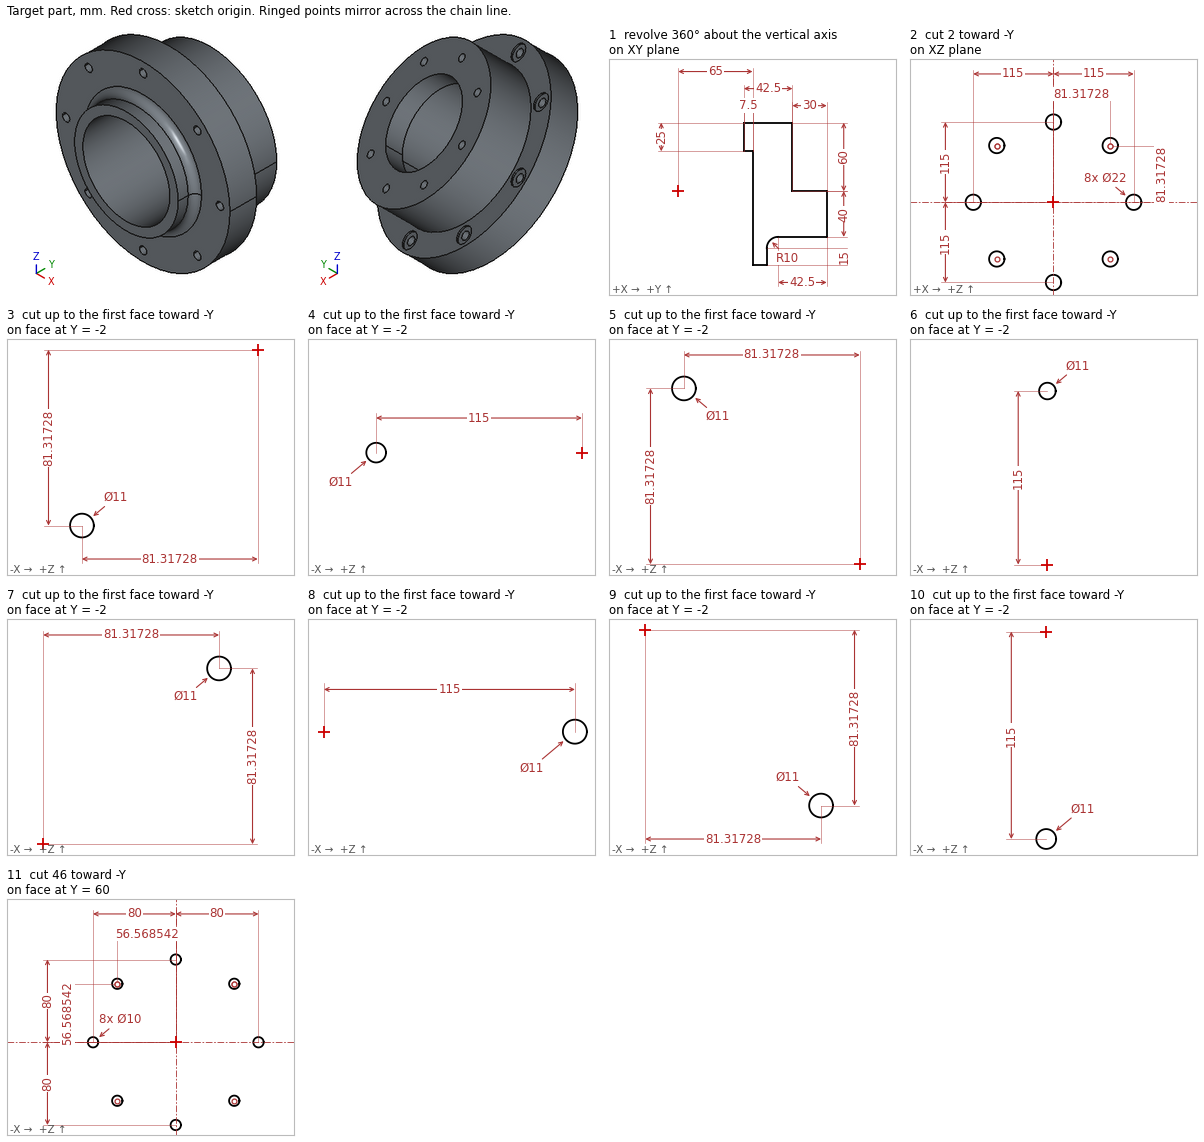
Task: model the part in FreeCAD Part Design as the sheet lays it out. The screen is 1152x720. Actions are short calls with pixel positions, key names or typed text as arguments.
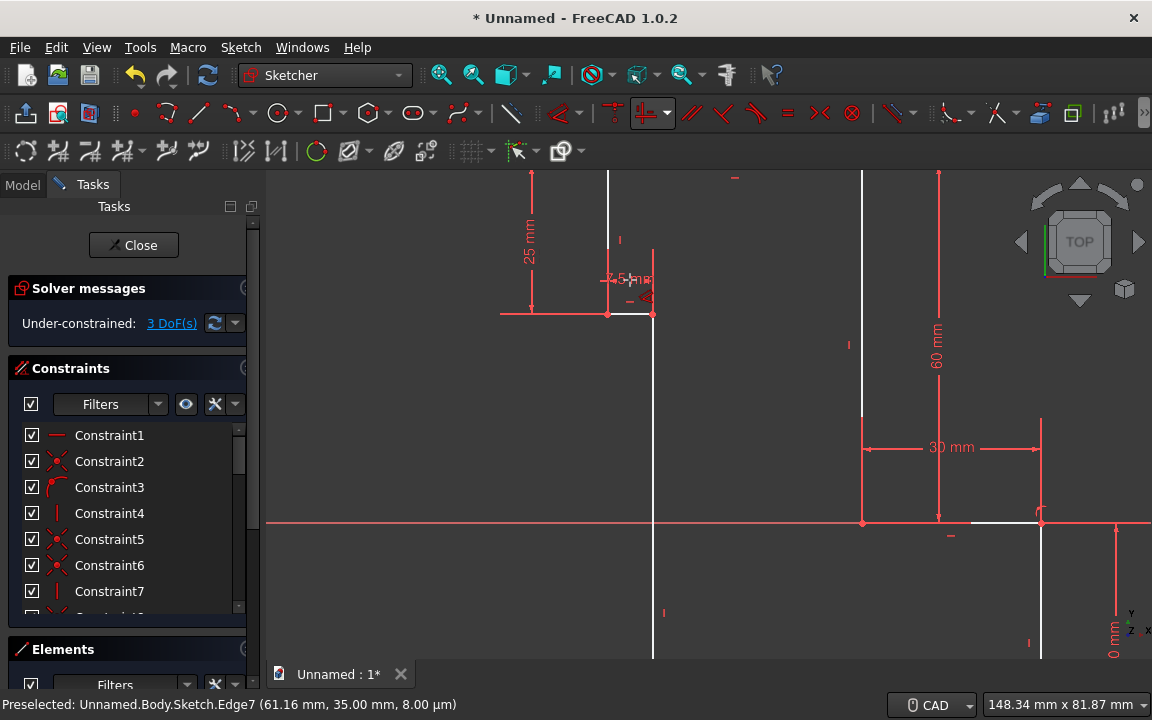
click(653, 314)
click(473, 280)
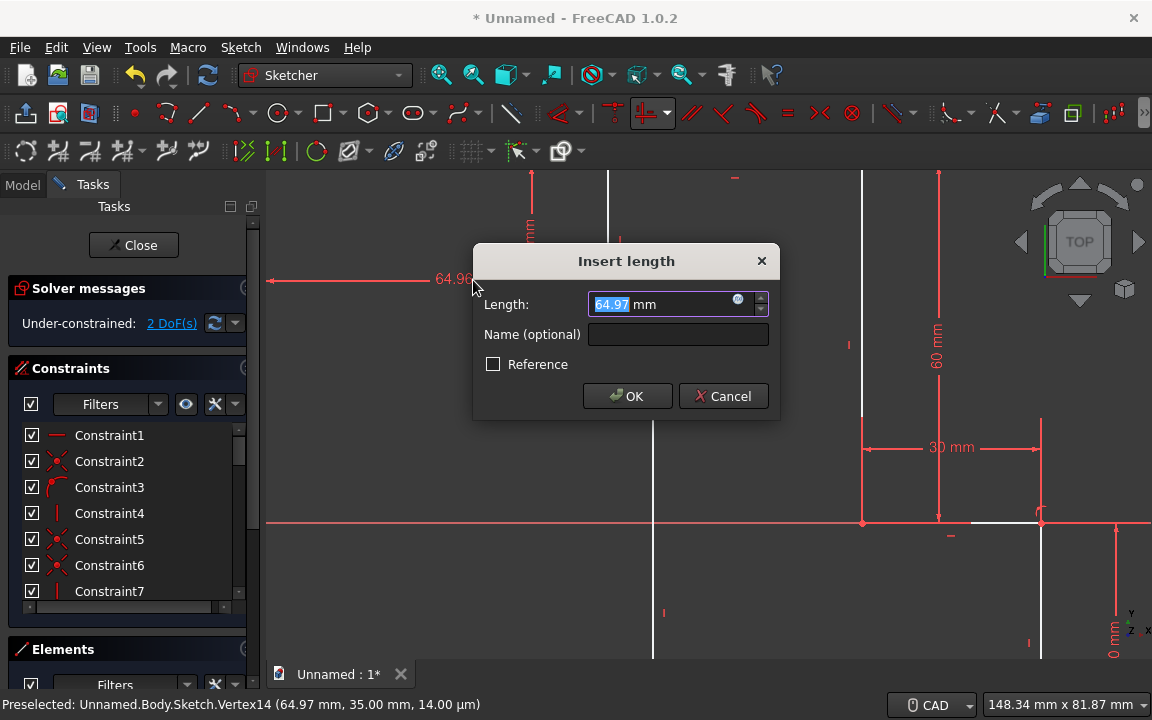
text(65)
key(Return)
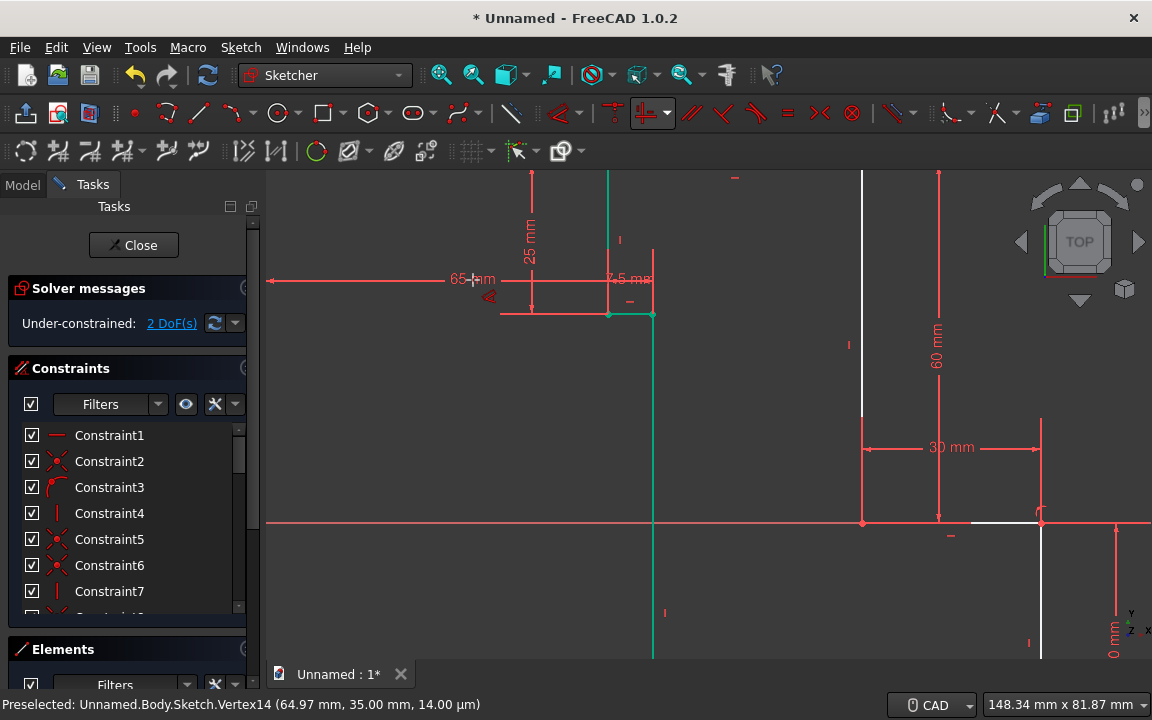
scroll(630, 314, down, 4)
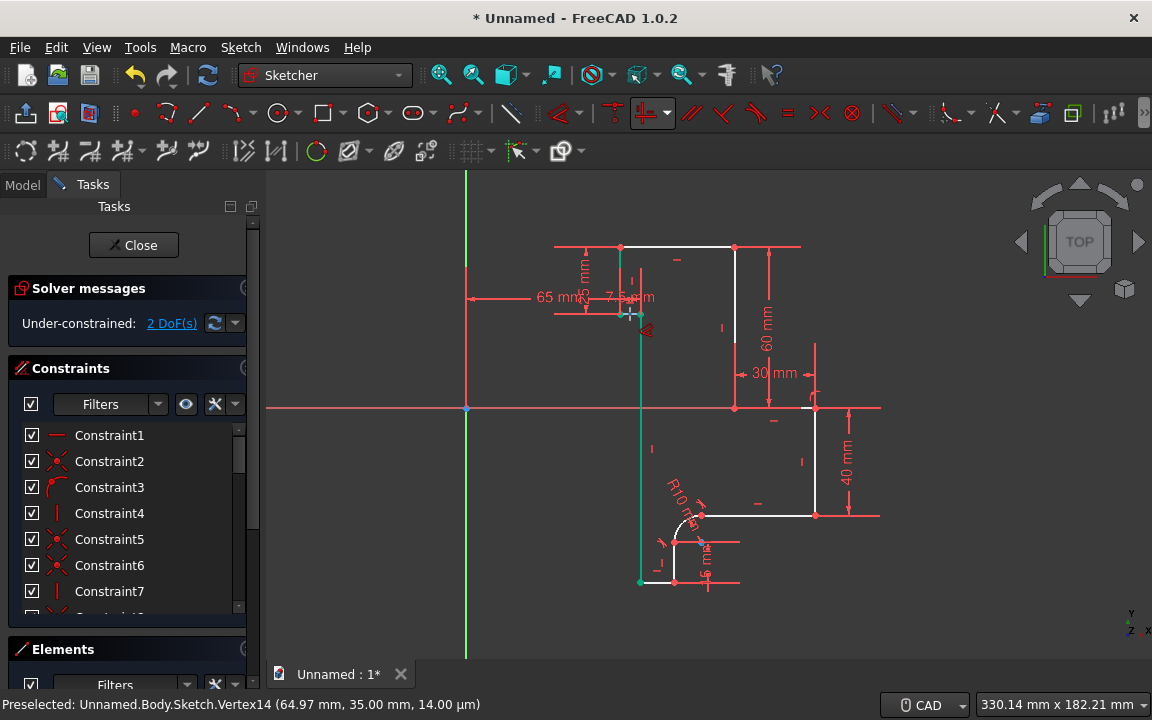
click(735, 516)
click(784, 550)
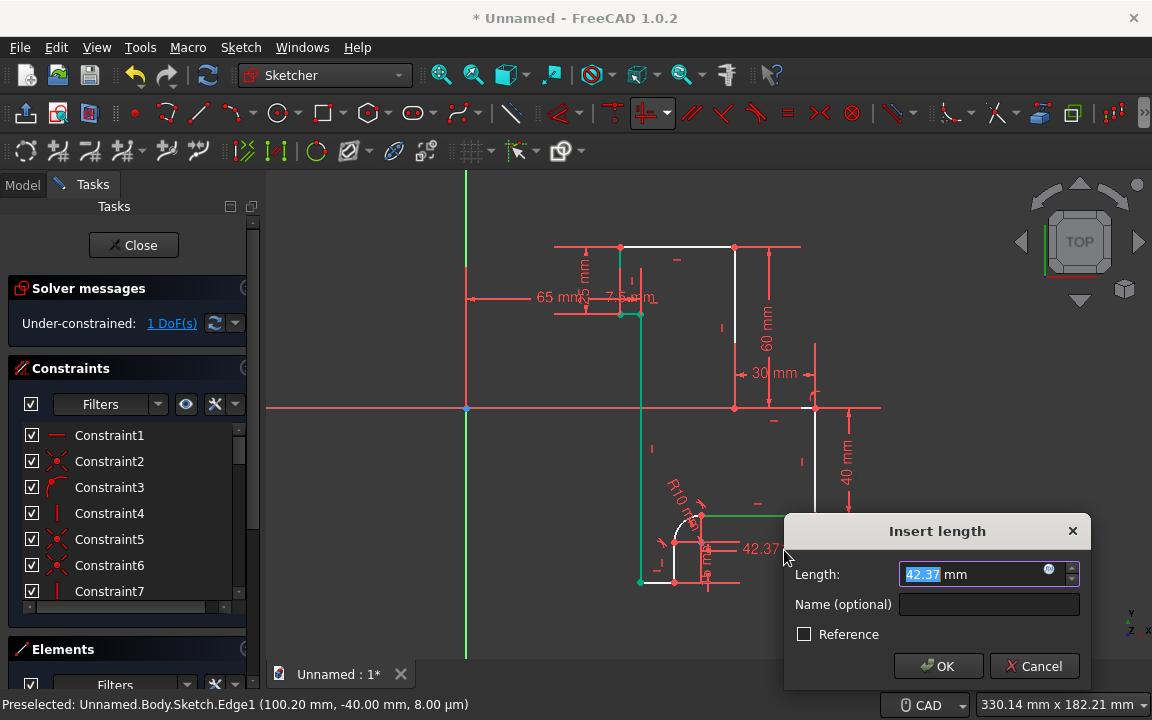
text(42.5)
key(Return)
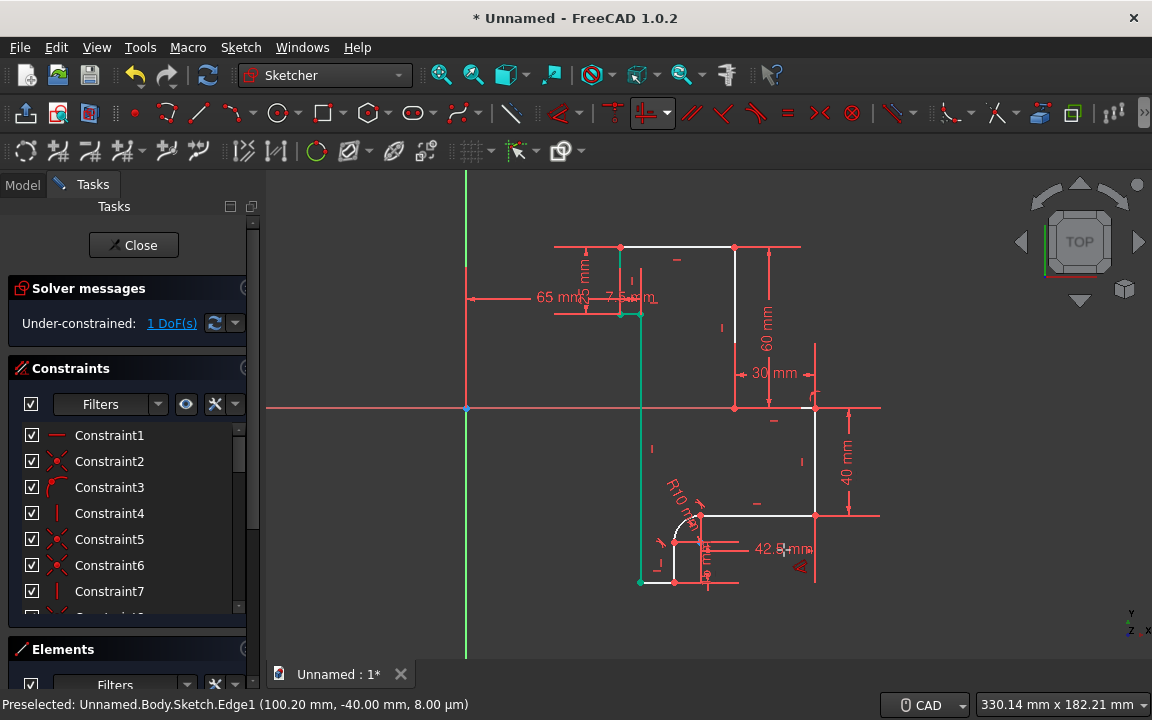
click(700, 247)
click(677, 213)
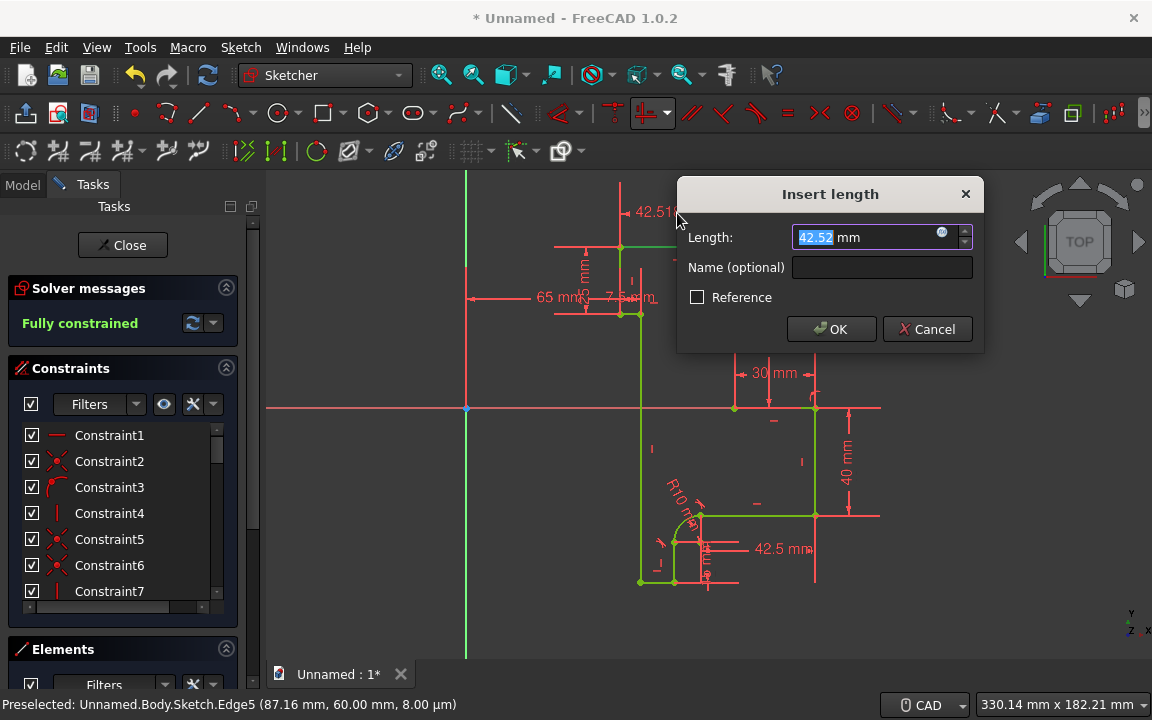
text(42.5)
key(Return)
key(Escape)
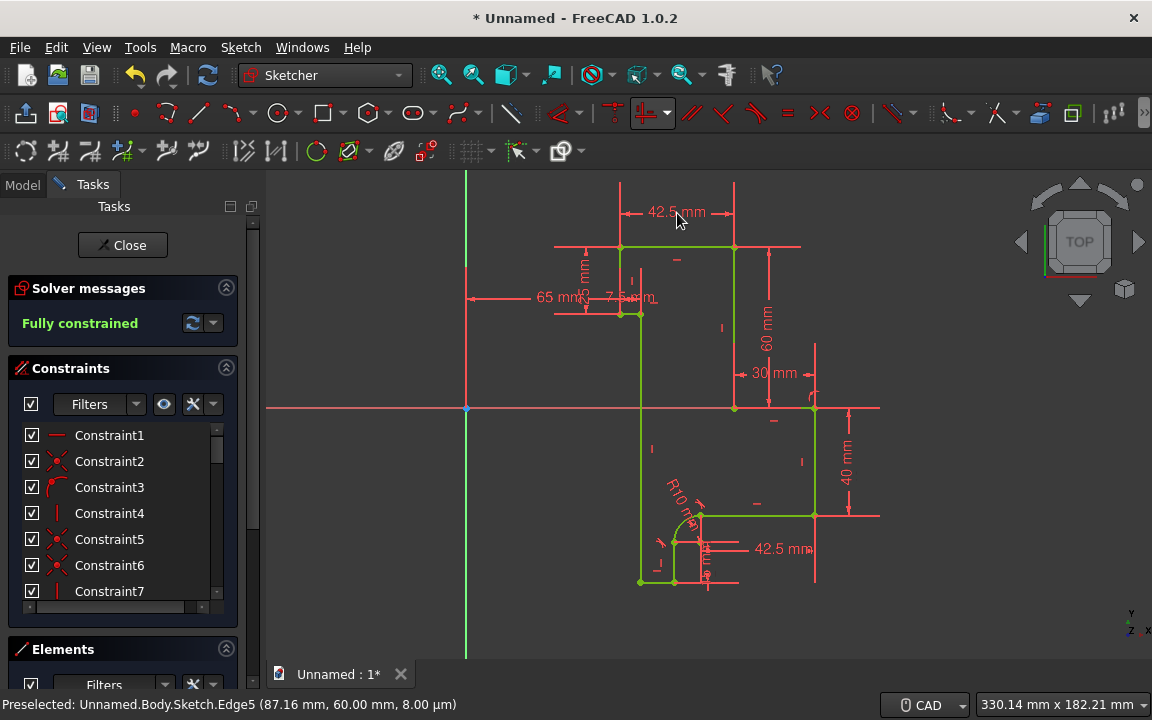
click(123, 245)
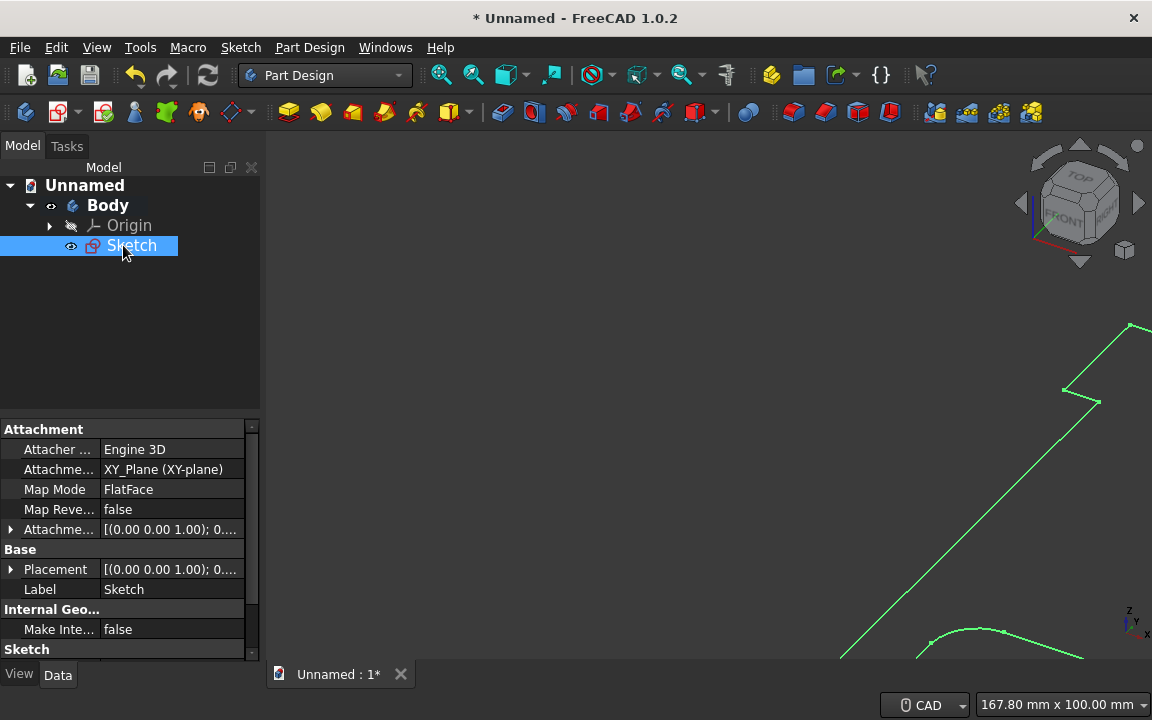
click(322, 112)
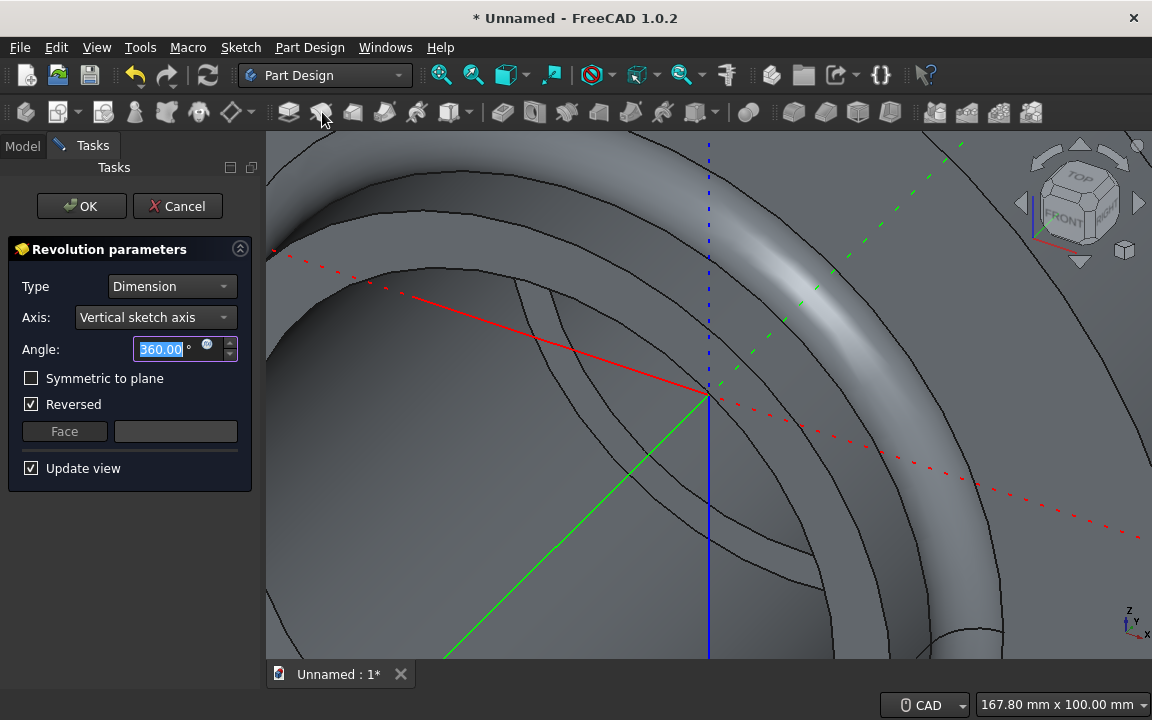
click(82, 206)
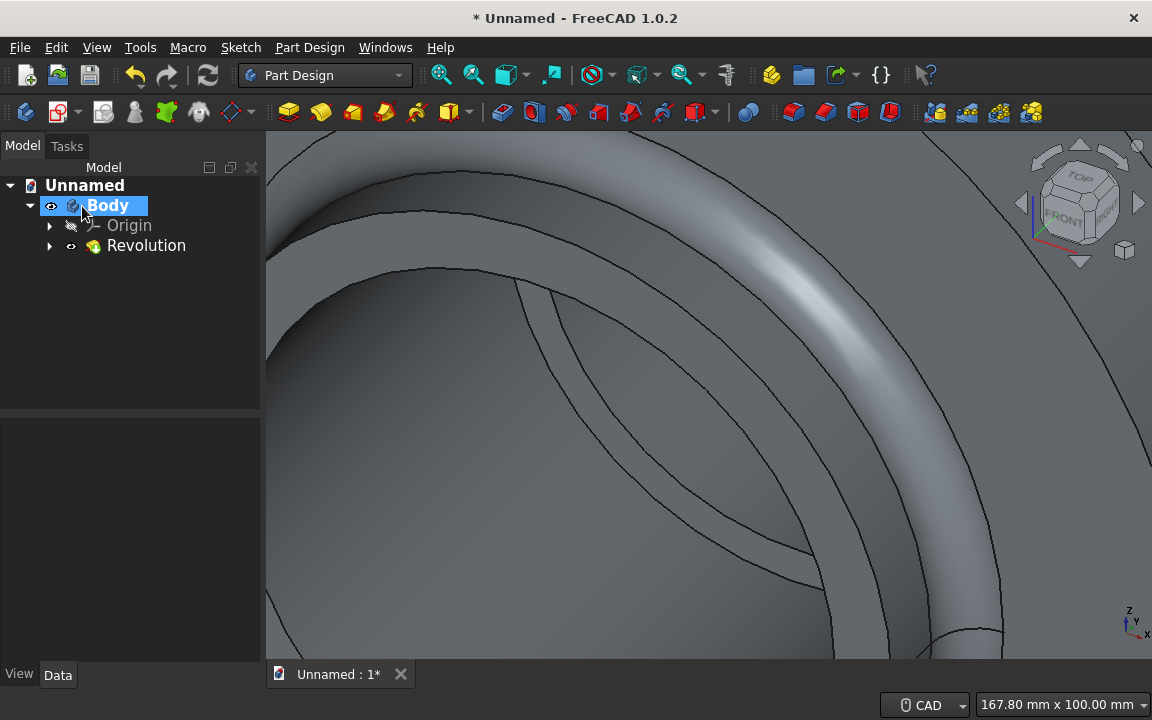
click(442, 76)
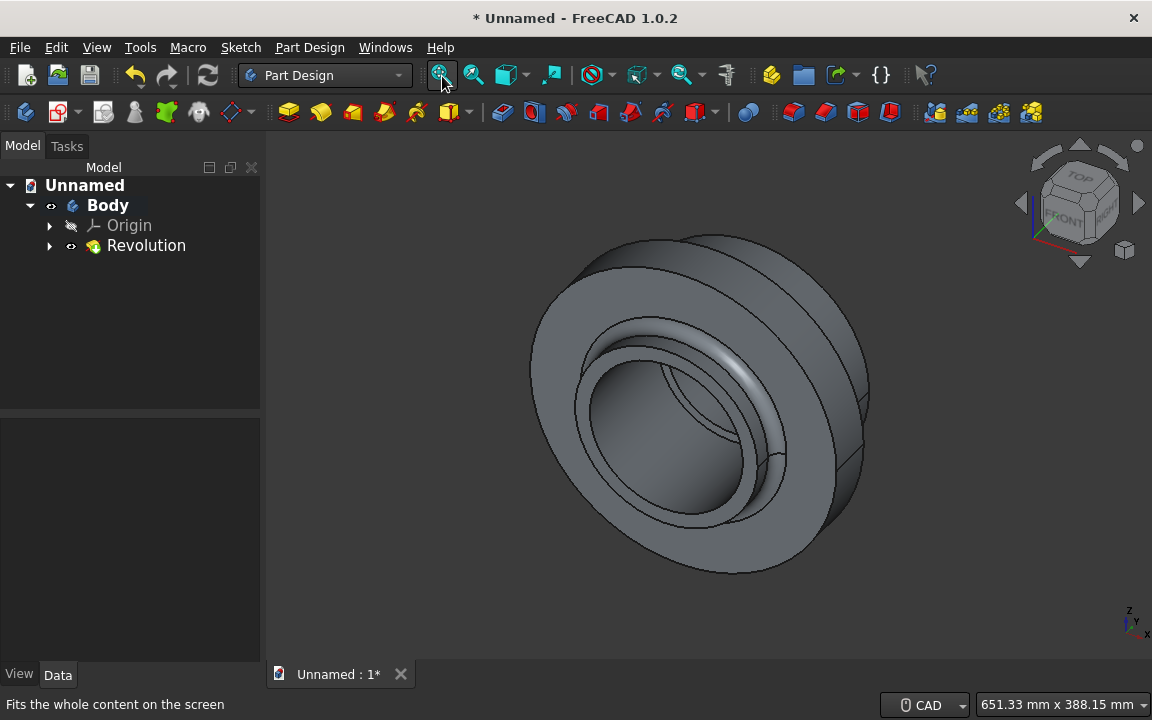
click(58, 112)